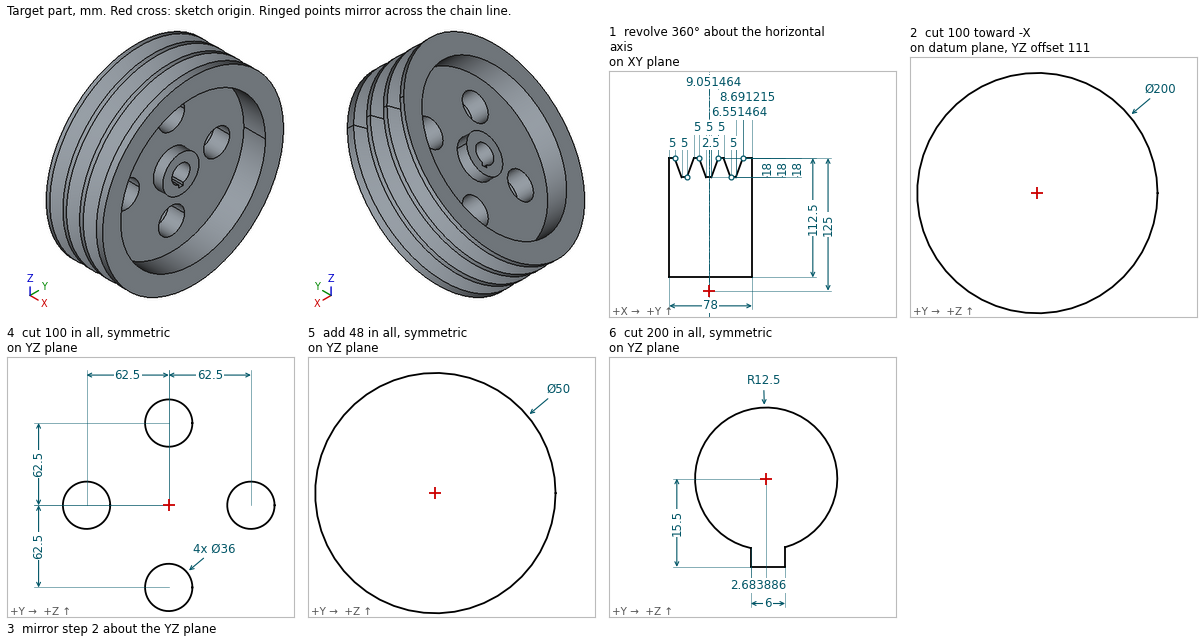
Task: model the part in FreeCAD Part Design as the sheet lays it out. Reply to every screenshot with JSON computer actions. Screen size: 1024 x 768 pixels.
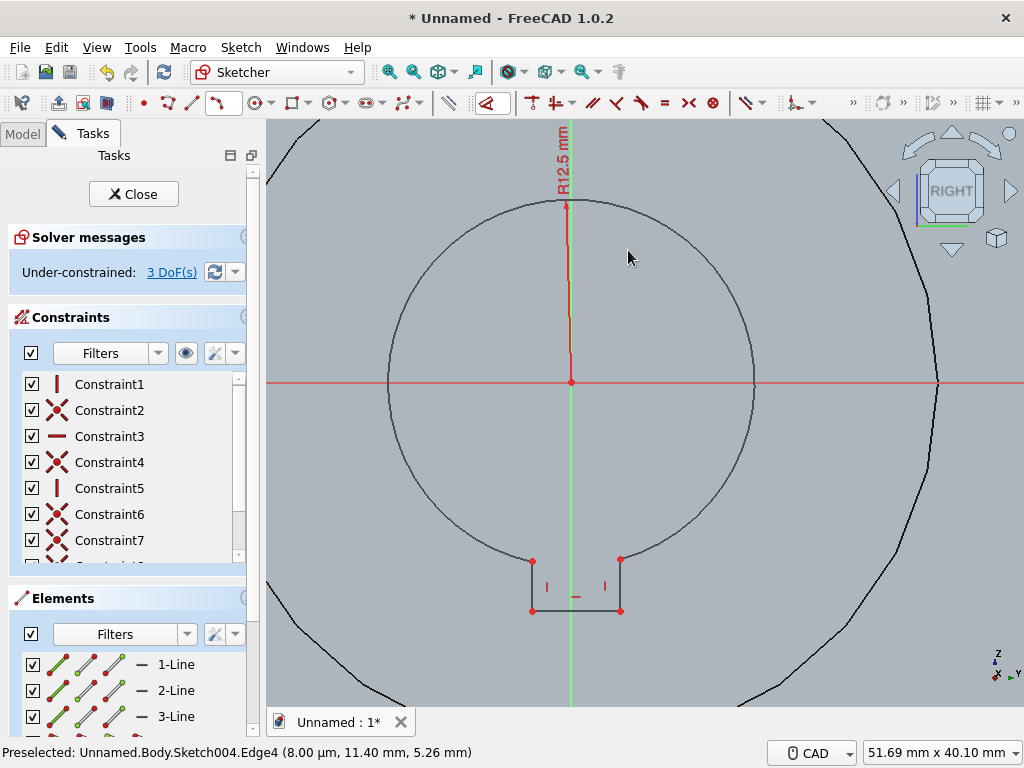
{"action": "left_click", "coordinate": [559, 611]}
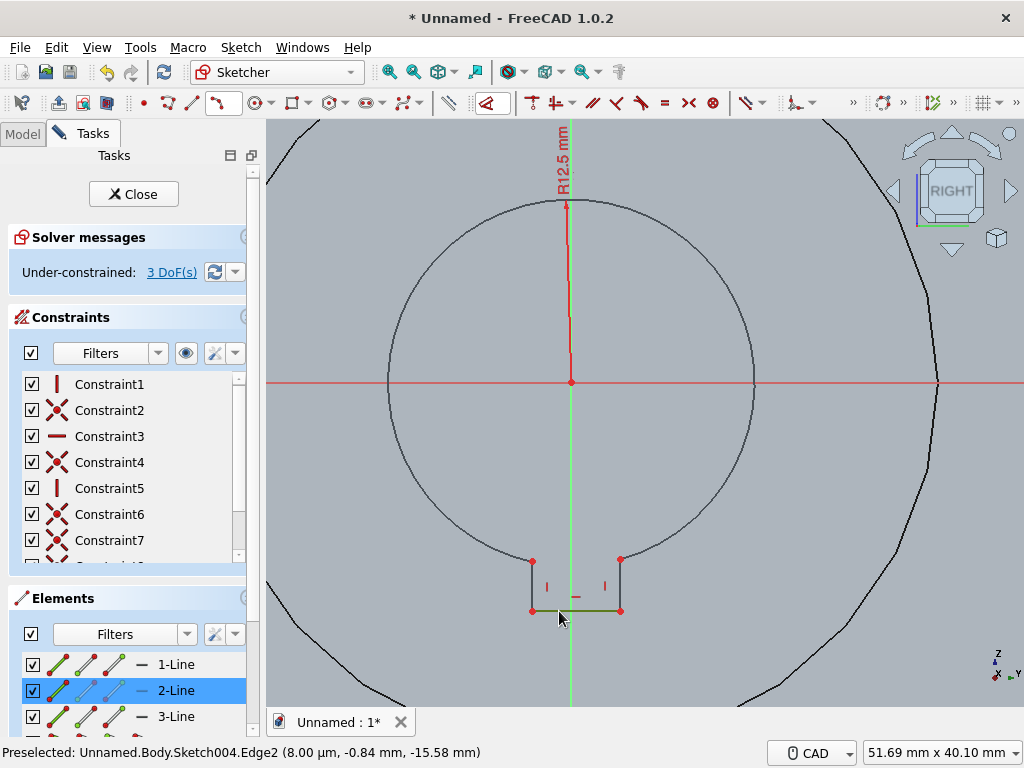
{"action": "key", "text": "l"}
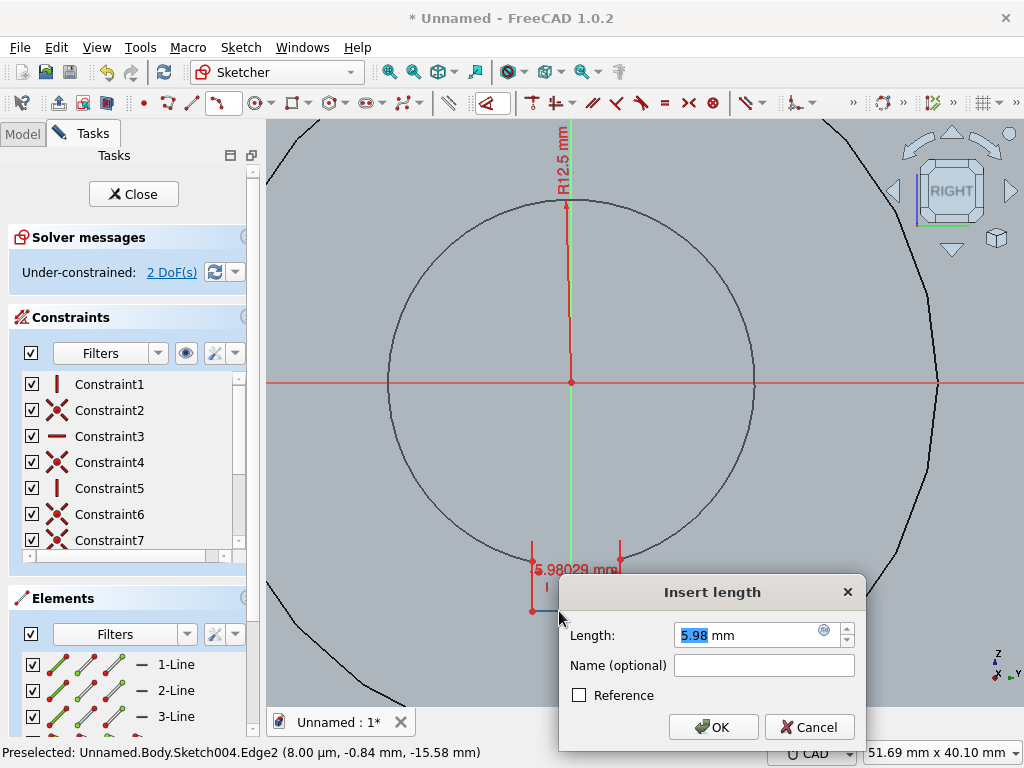
{"action": "type", "text": "6"}
{"action": "key", "text": "Return"}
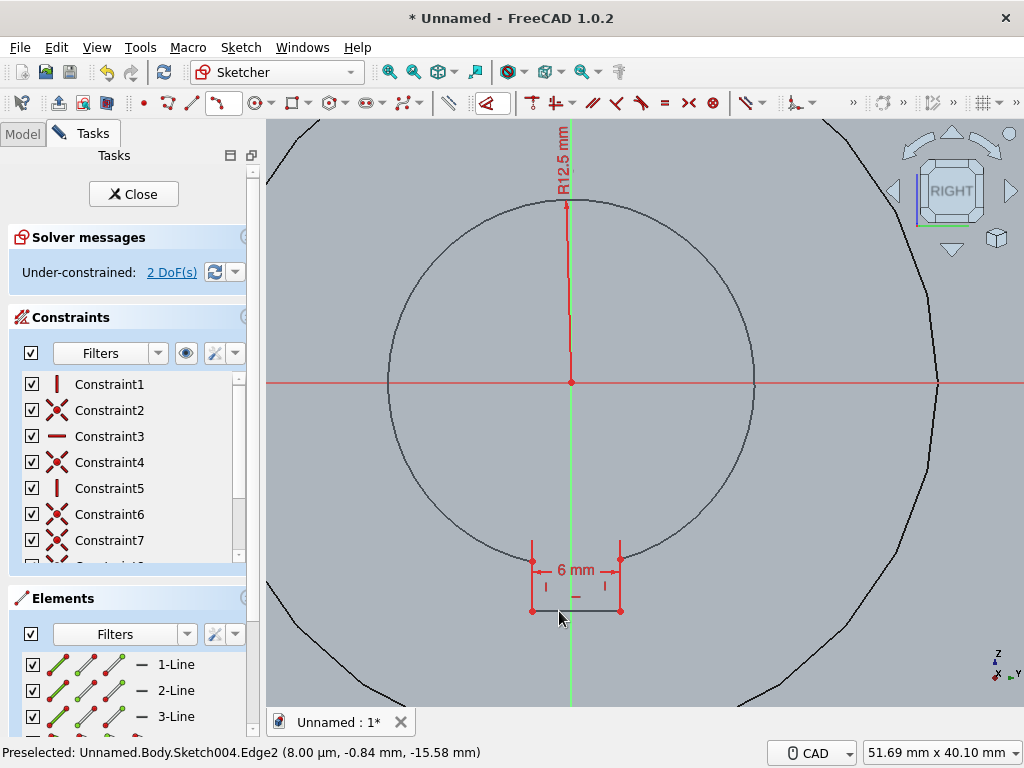
{"action": "left_click", "coordinate": [532, 611]}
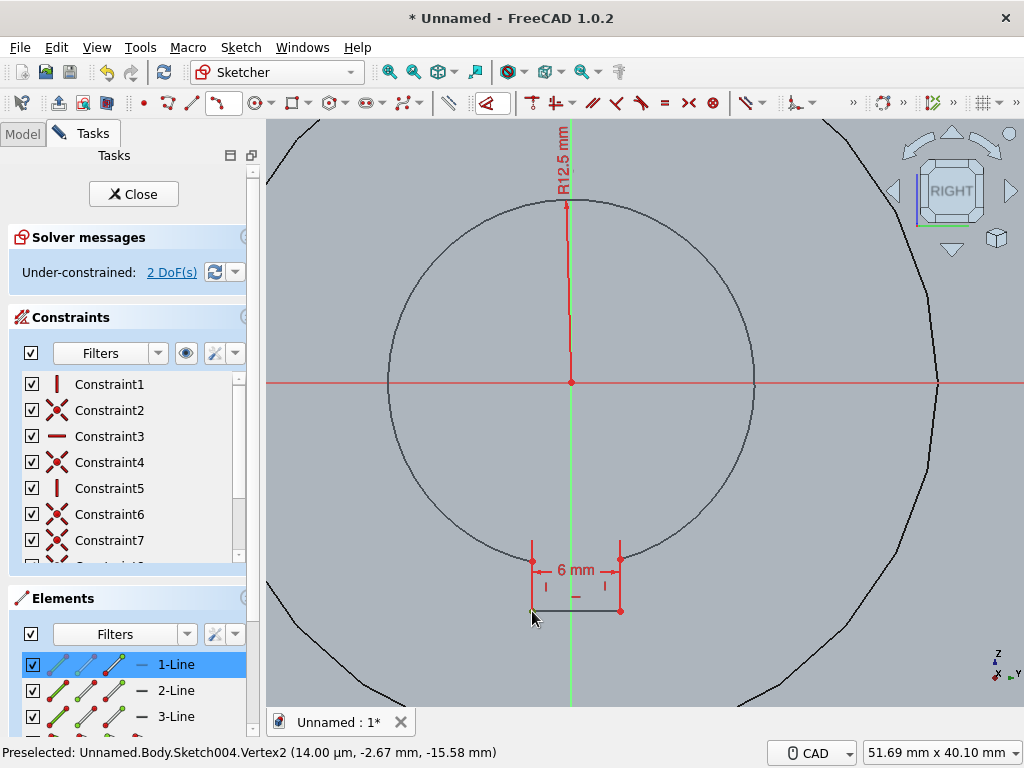
{"action": "key", "text": "i"}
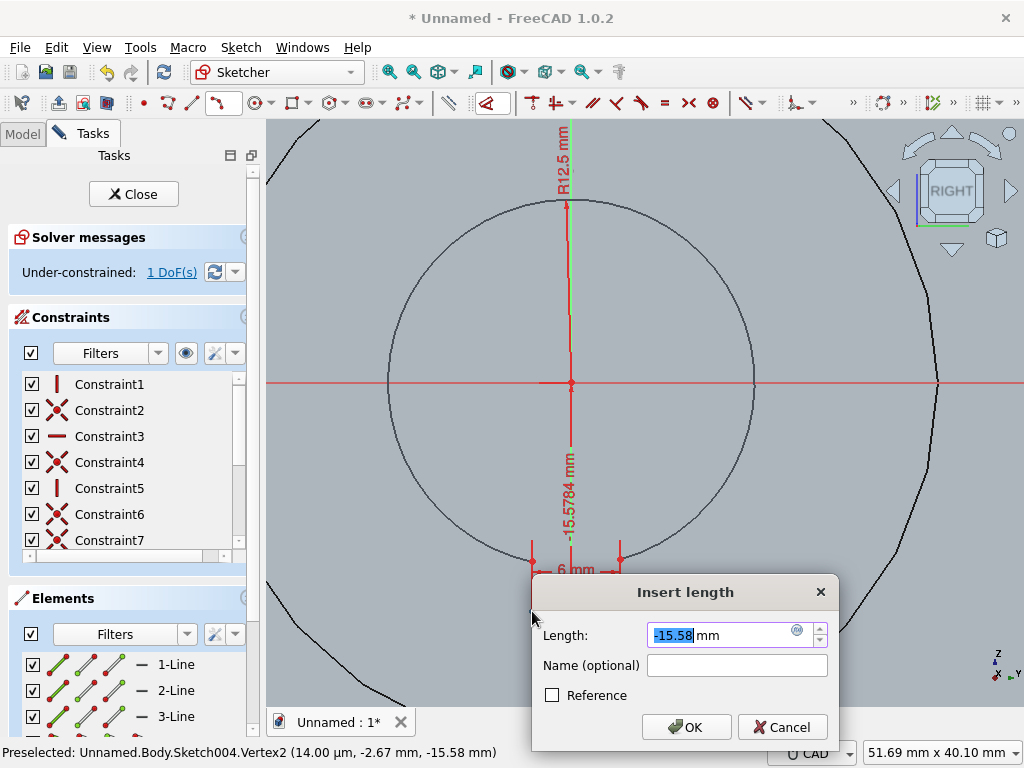
{"action": "type", "text": "-15.5"}
{"action": "key", "text": "Return"}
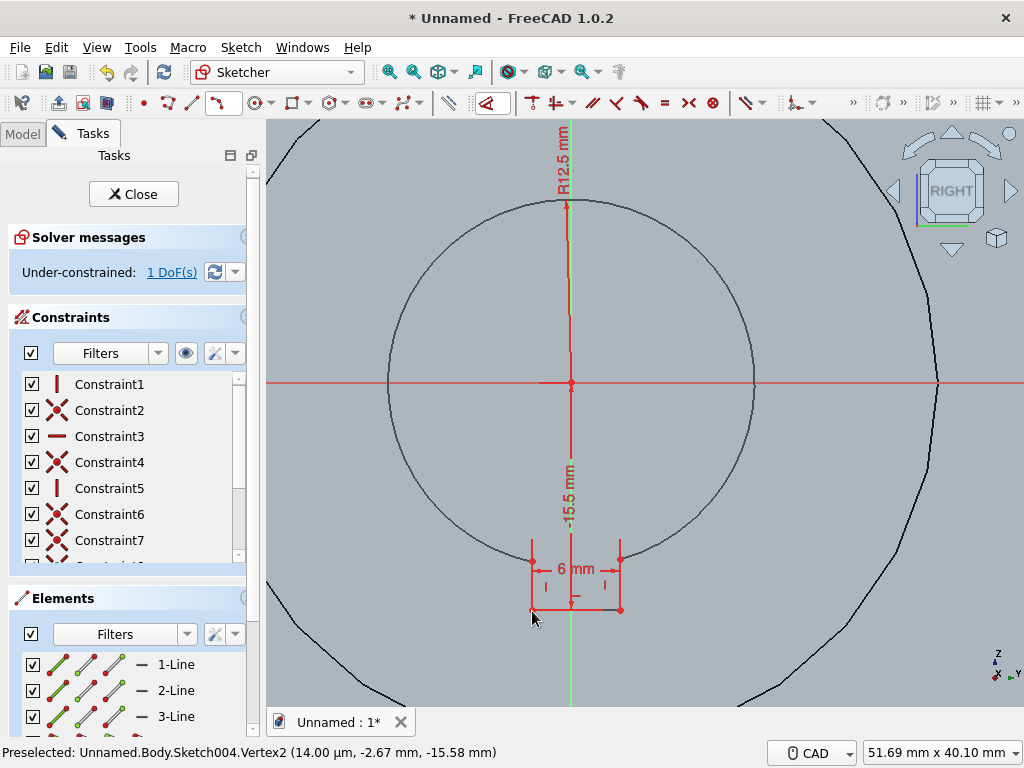
{"action": "left_click", "coordinate": [532, 562]}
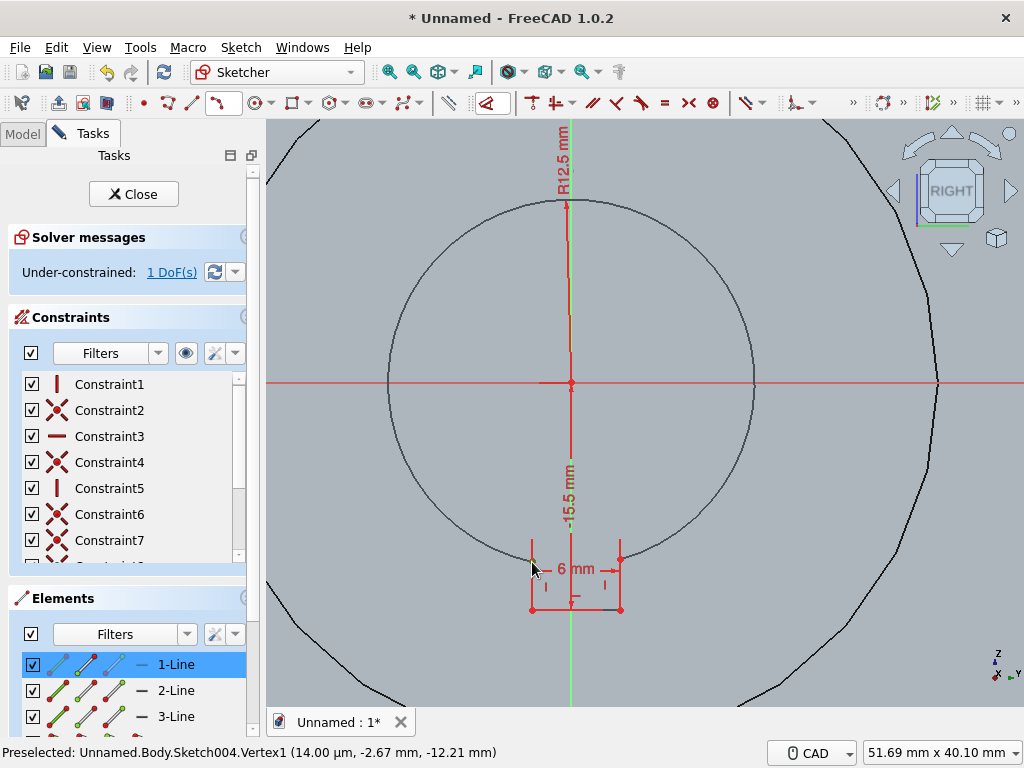
{"action": "key", "text": "l"}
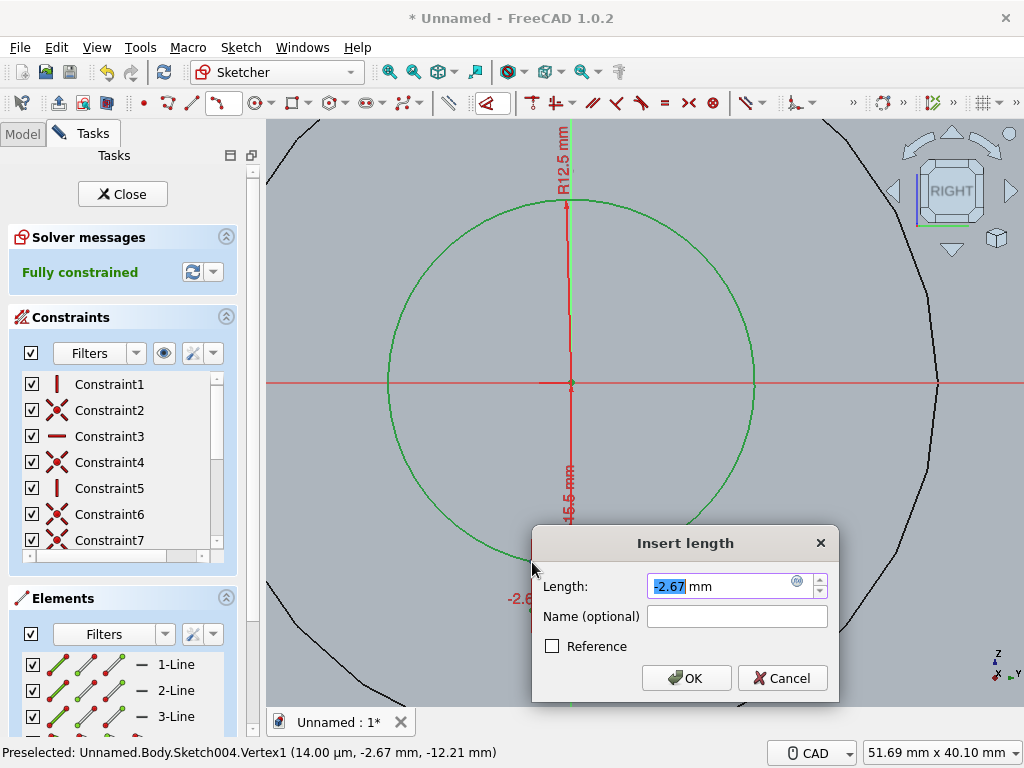
{"action": "type", "text": "-2.683886"}
{"action": "key", "text": "Return"}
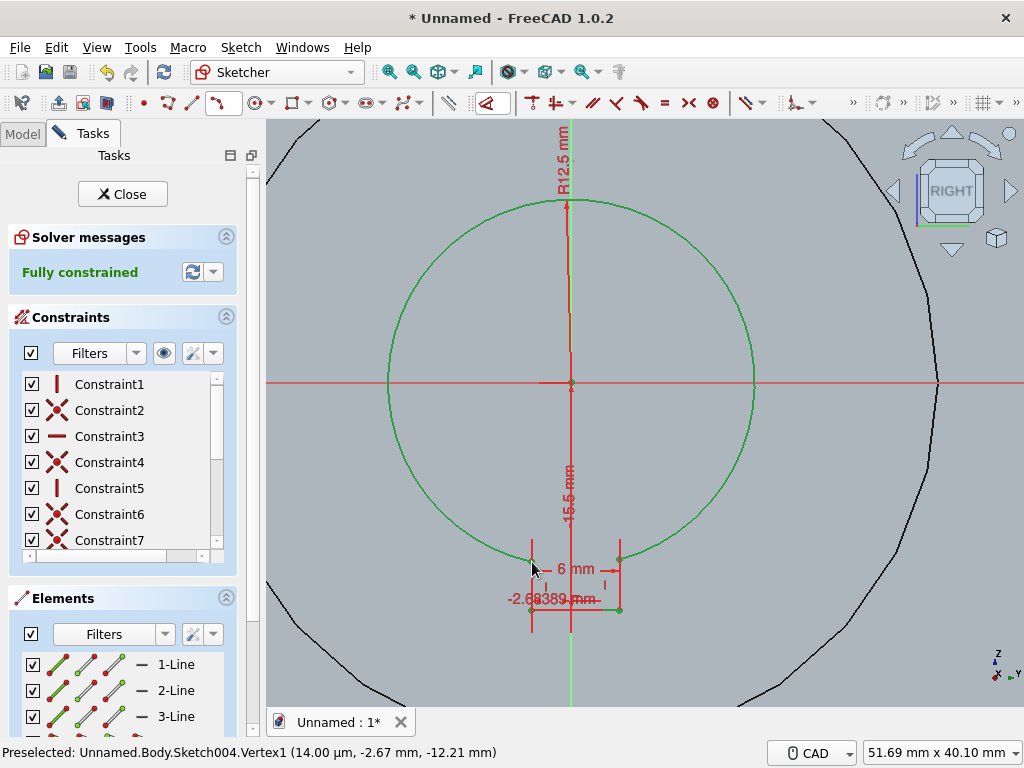
{"action": "left_click", "coordinate": [123, 194]}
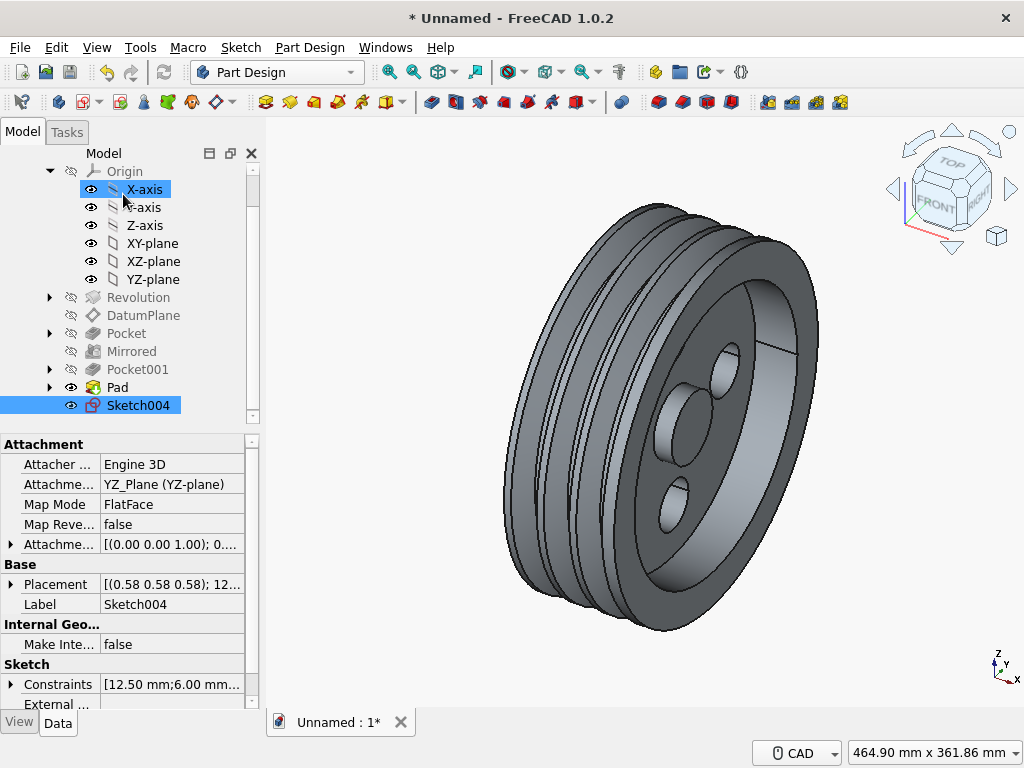
{"action": "left_click", "coordinate": [432, 102]}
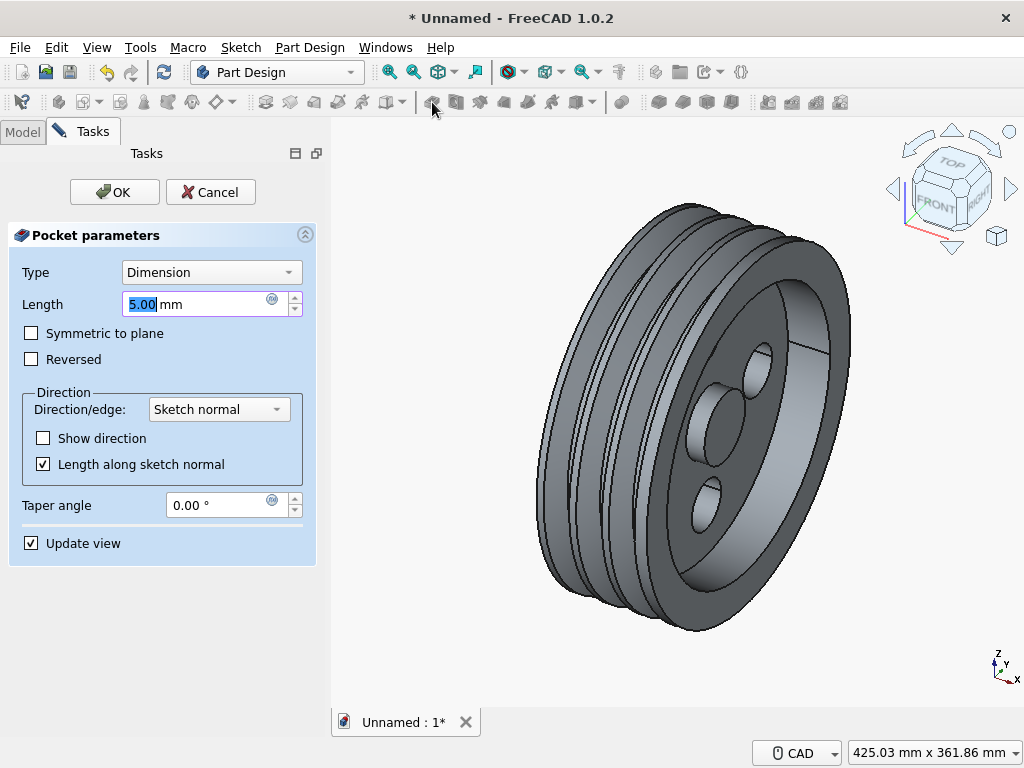
{"action": "type", "text": "200"}
{"action": "key", "text": "Tab"}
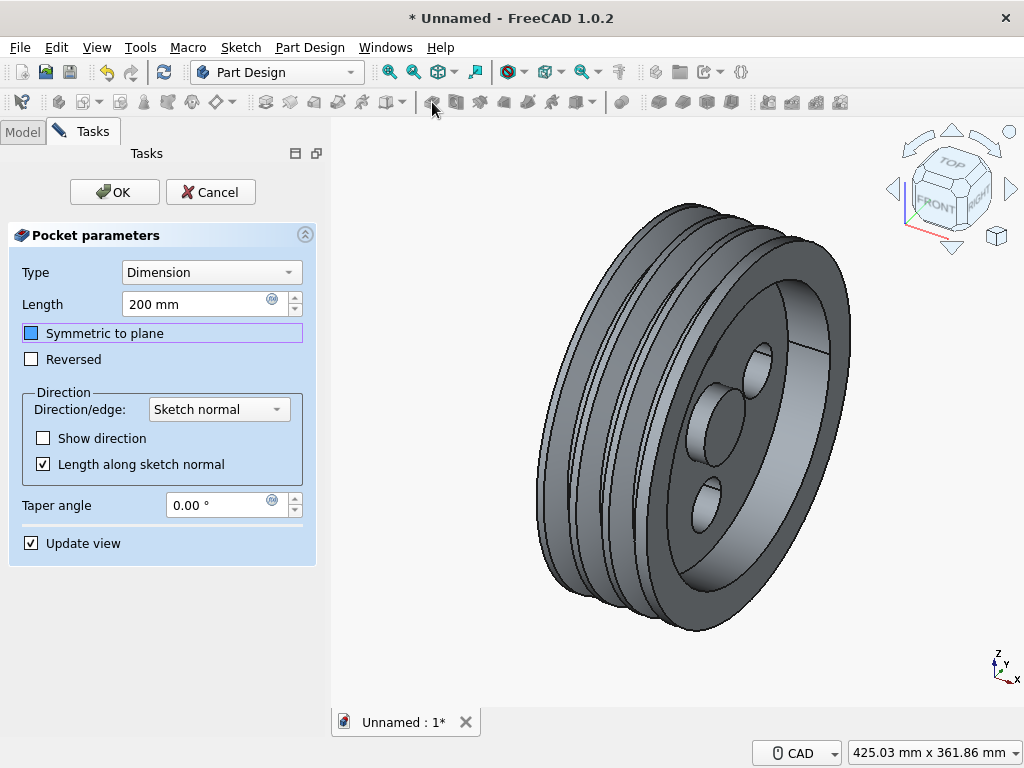
{"action": "left_click", "coordinate": [30, 333]}